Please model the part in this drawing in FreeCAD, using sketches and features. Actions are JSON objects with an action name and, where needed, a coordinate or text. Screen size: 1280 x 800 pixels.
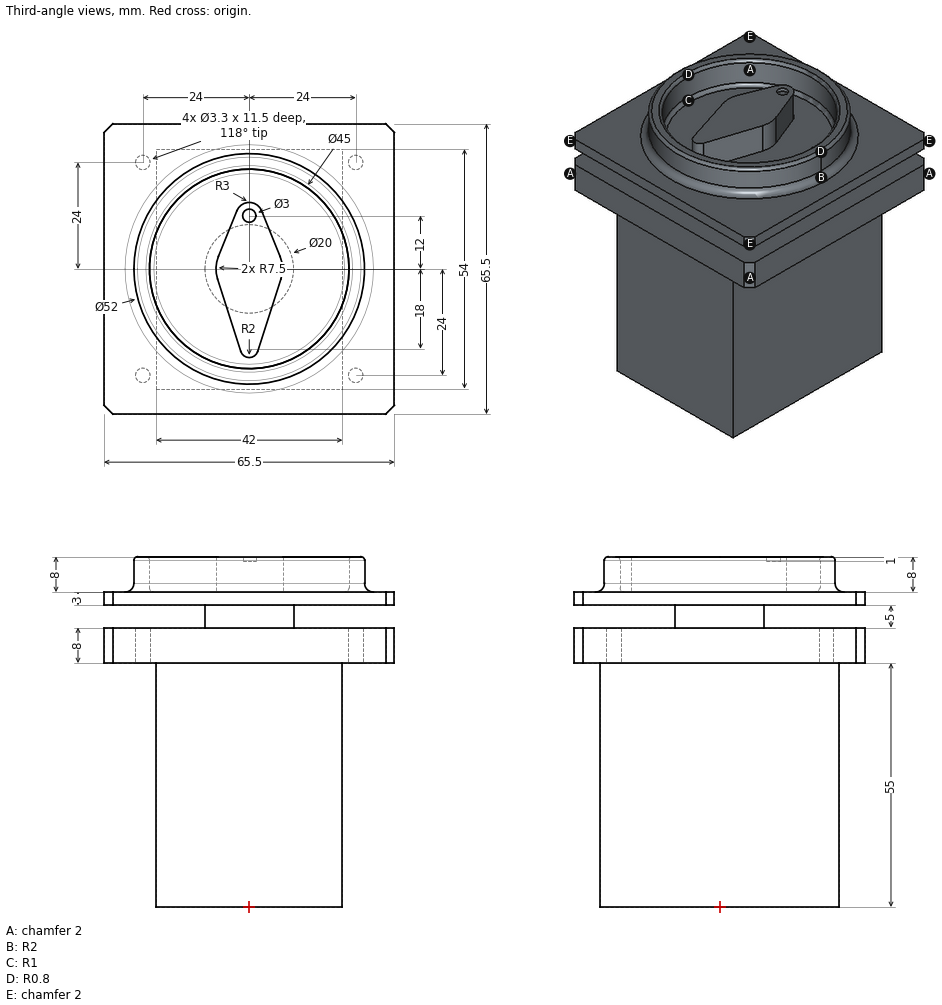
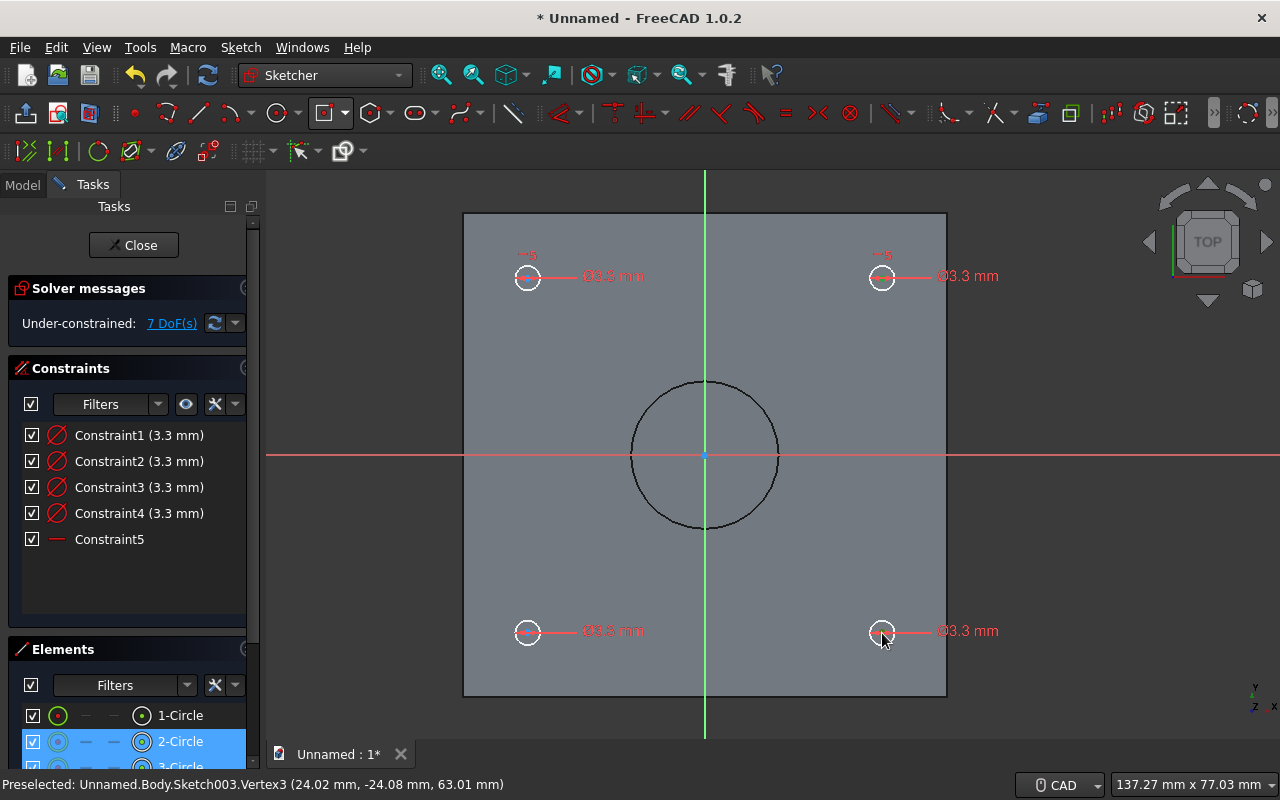
{"action": "left_click", "coordinate": [668, 114]}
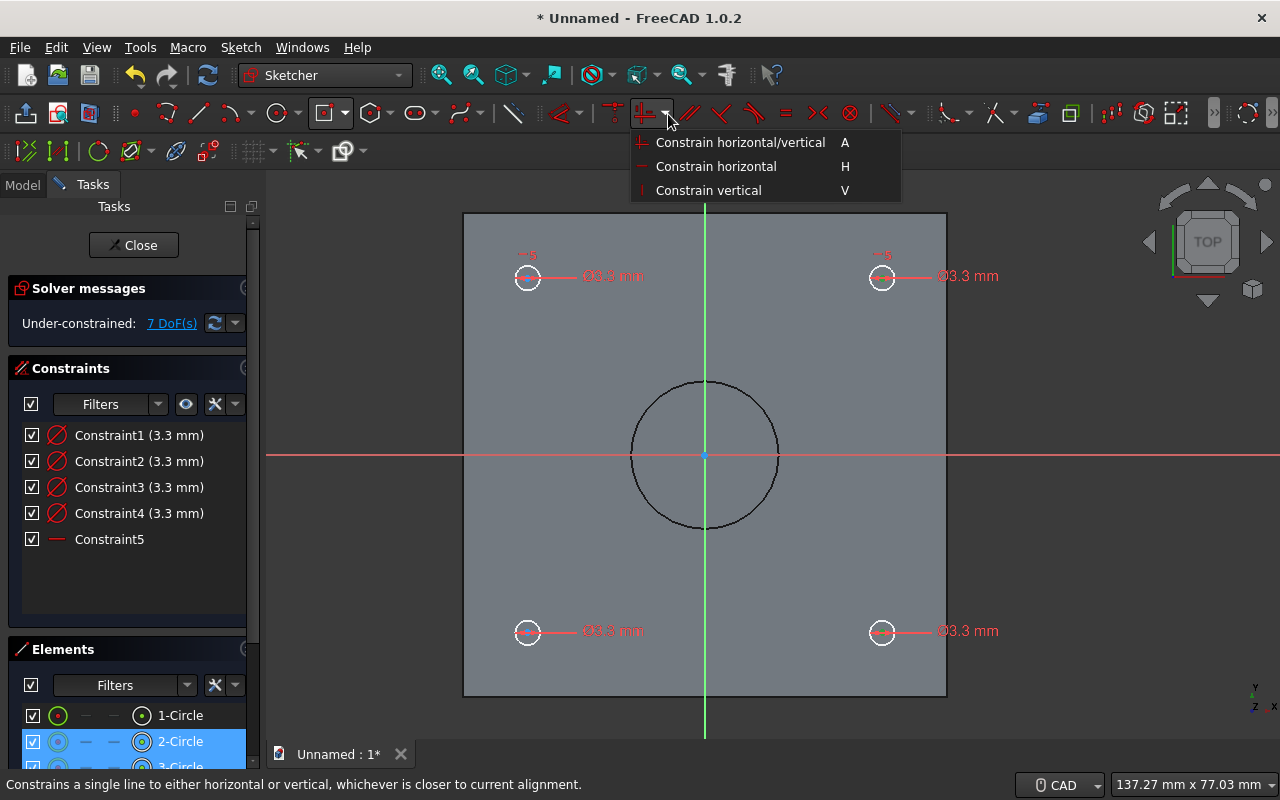
{"action": "left_click", "coordinate": [766, 190]}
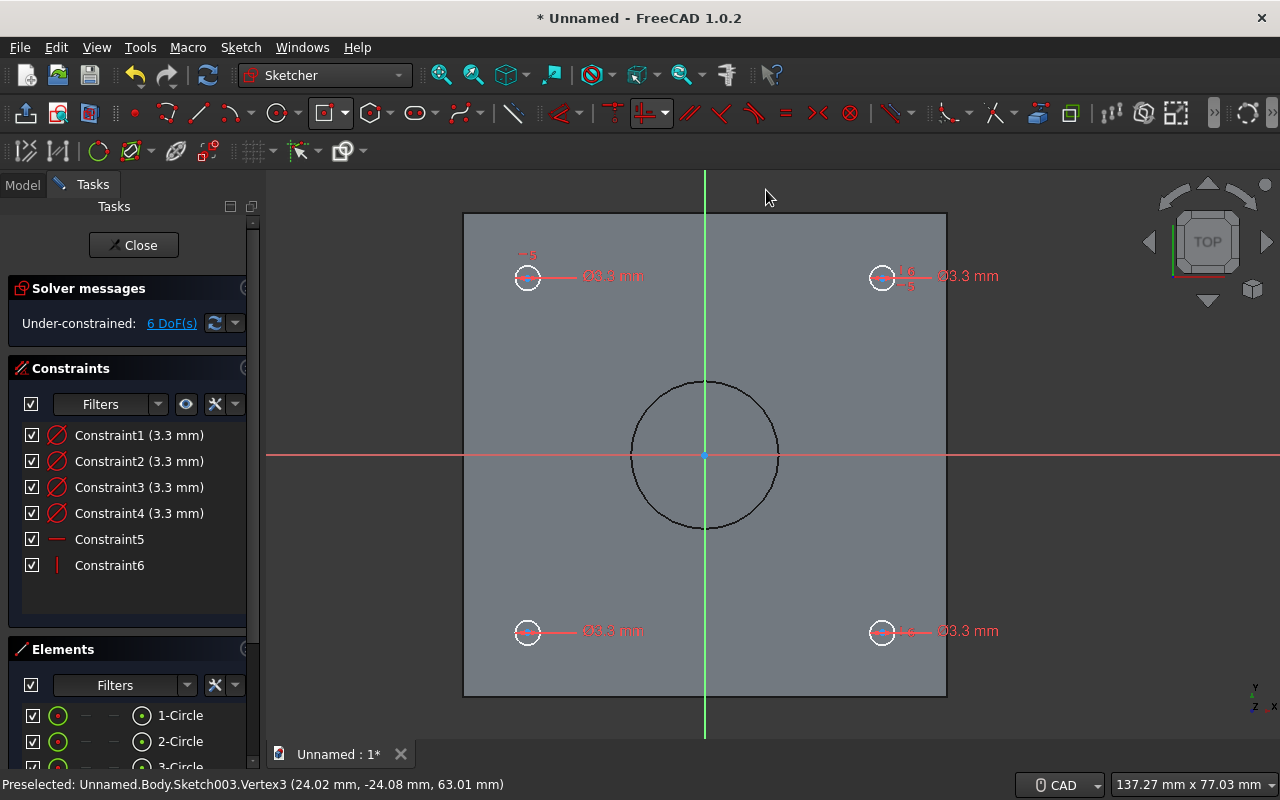
{"action": "left_click", "coordinate": [528, 278]}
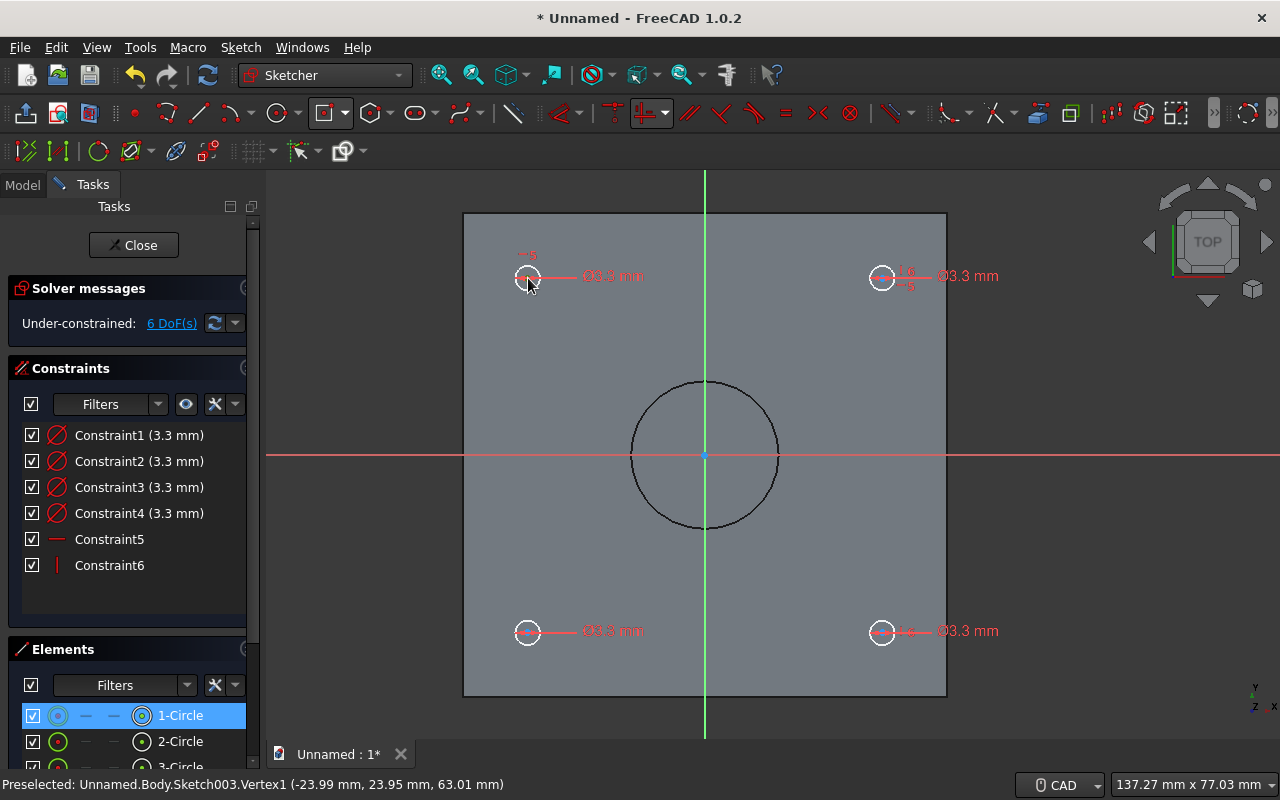
{"action": "left_click", "coordinate": [528, 633]}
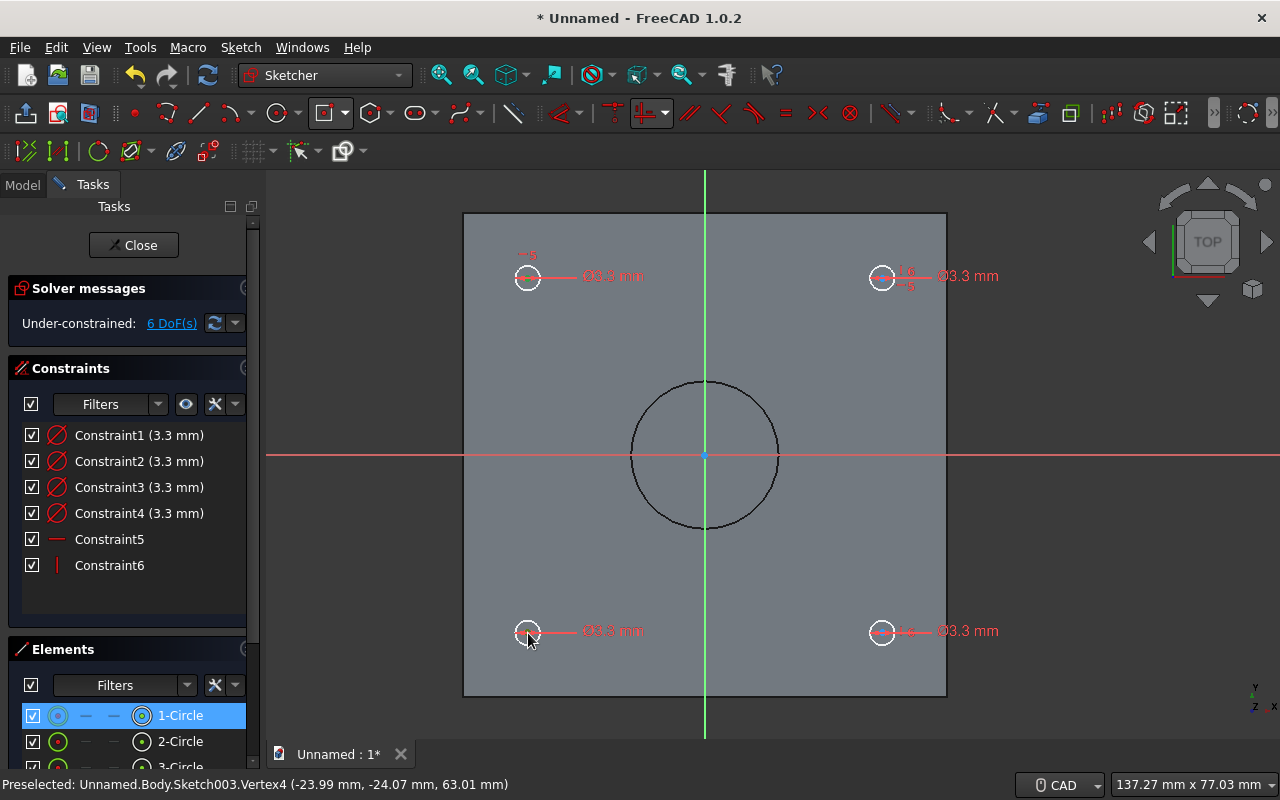
{"action": "key", "text": "v"}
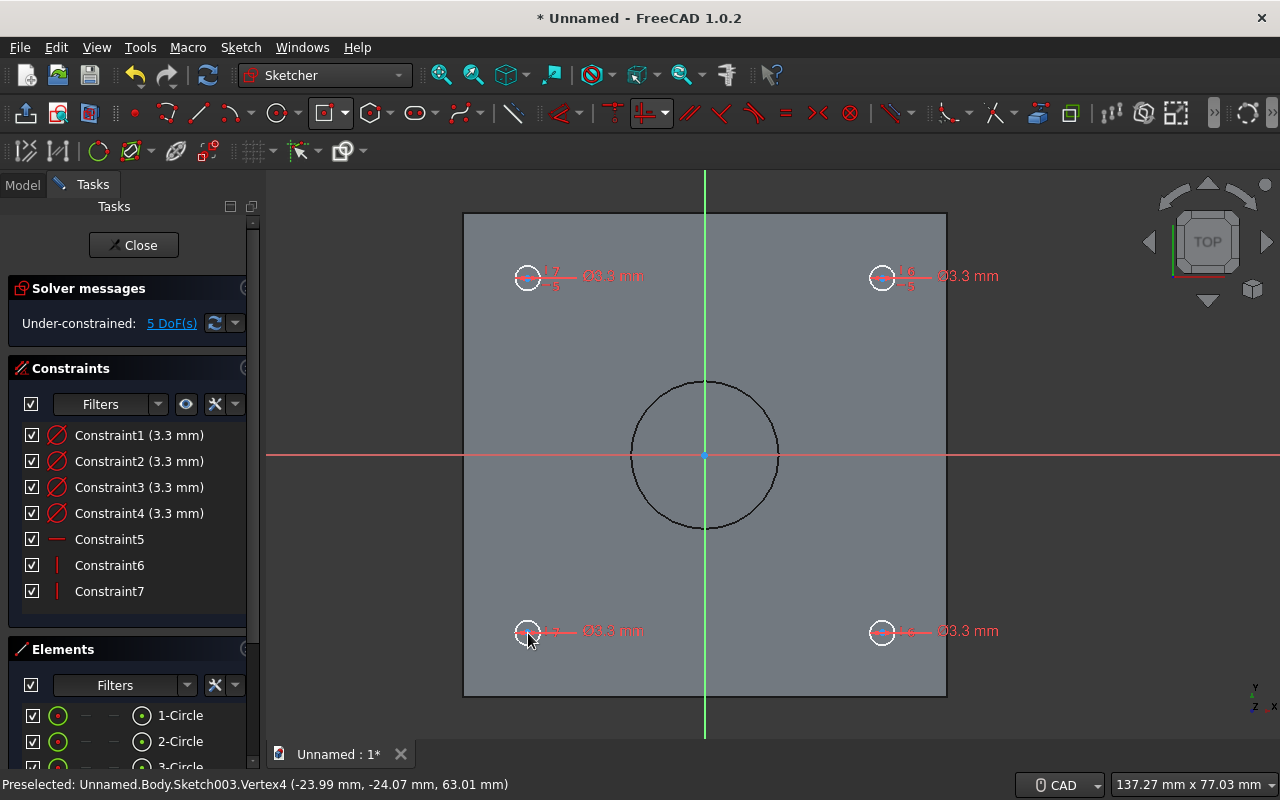
{"action": "left_click", "coordinate": [882, 633]}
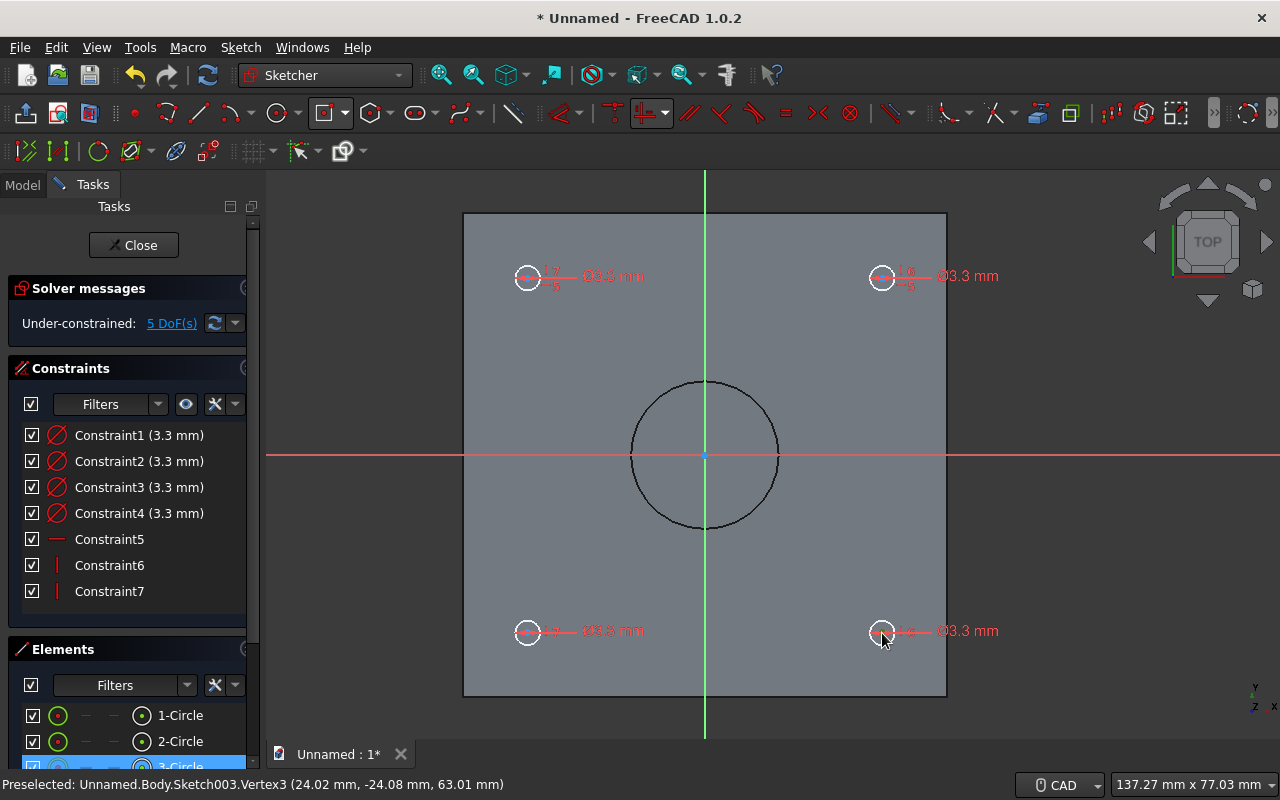
{"action": "left_click", "coordinate": [528, 633]}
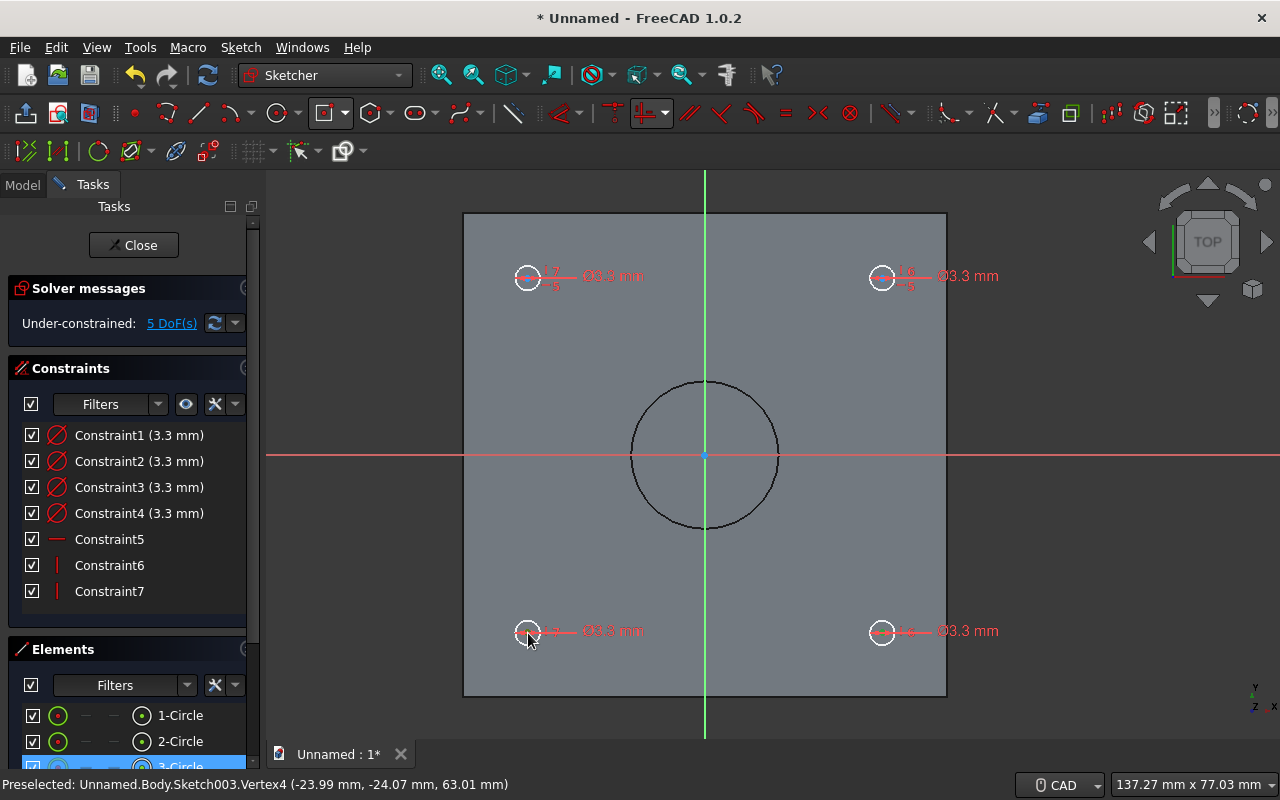
{"action": "key", "text": "h"}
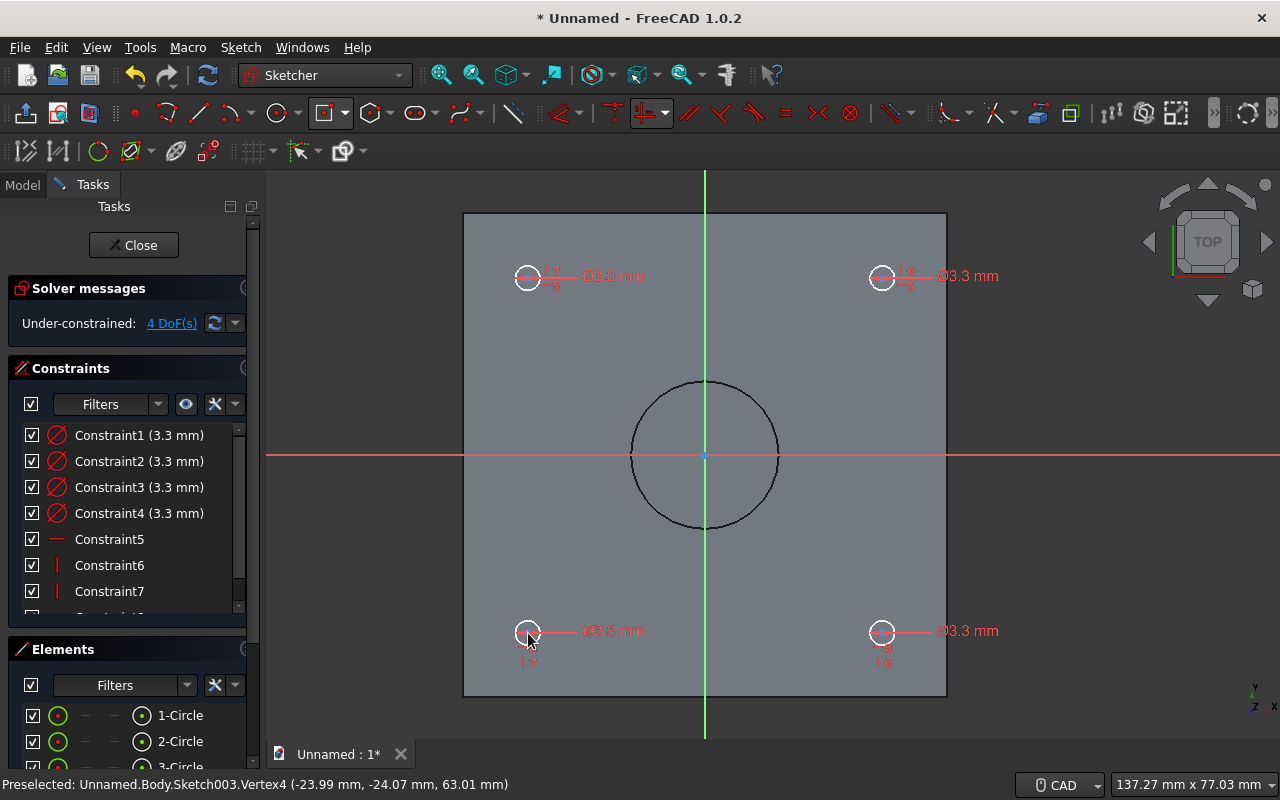
{"action": "left_click", "coordinate": [560, 114]}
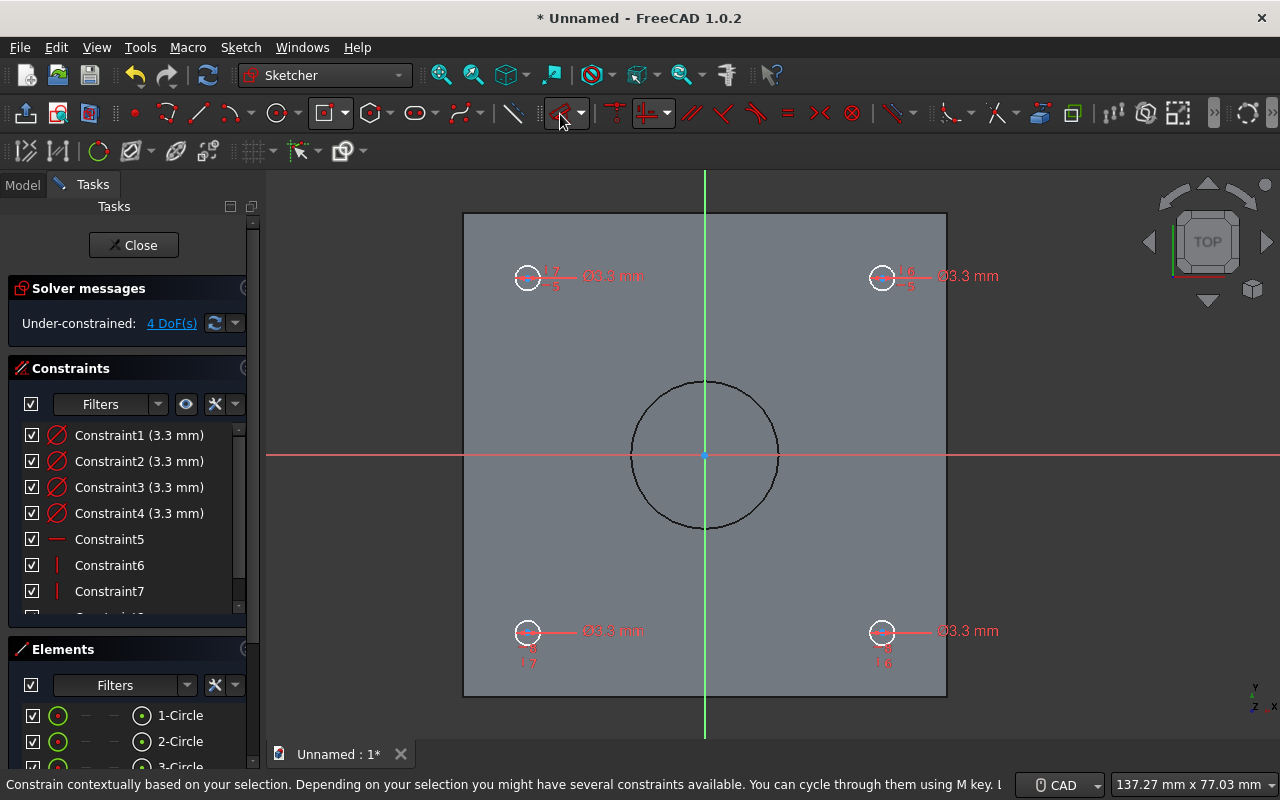
{"action": "left_click", "coordinate": [528, 278]}
{"action": "left_click", "coordinate": [616, 244]}